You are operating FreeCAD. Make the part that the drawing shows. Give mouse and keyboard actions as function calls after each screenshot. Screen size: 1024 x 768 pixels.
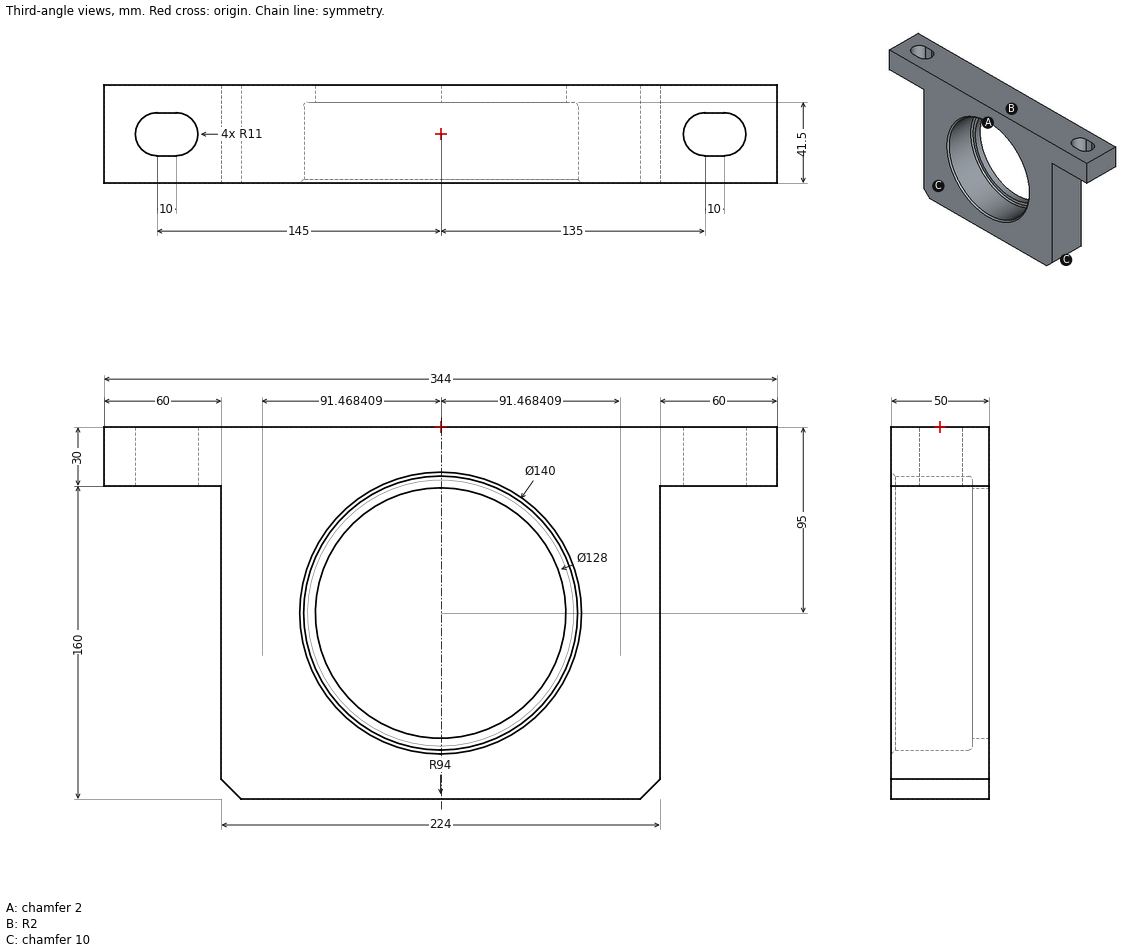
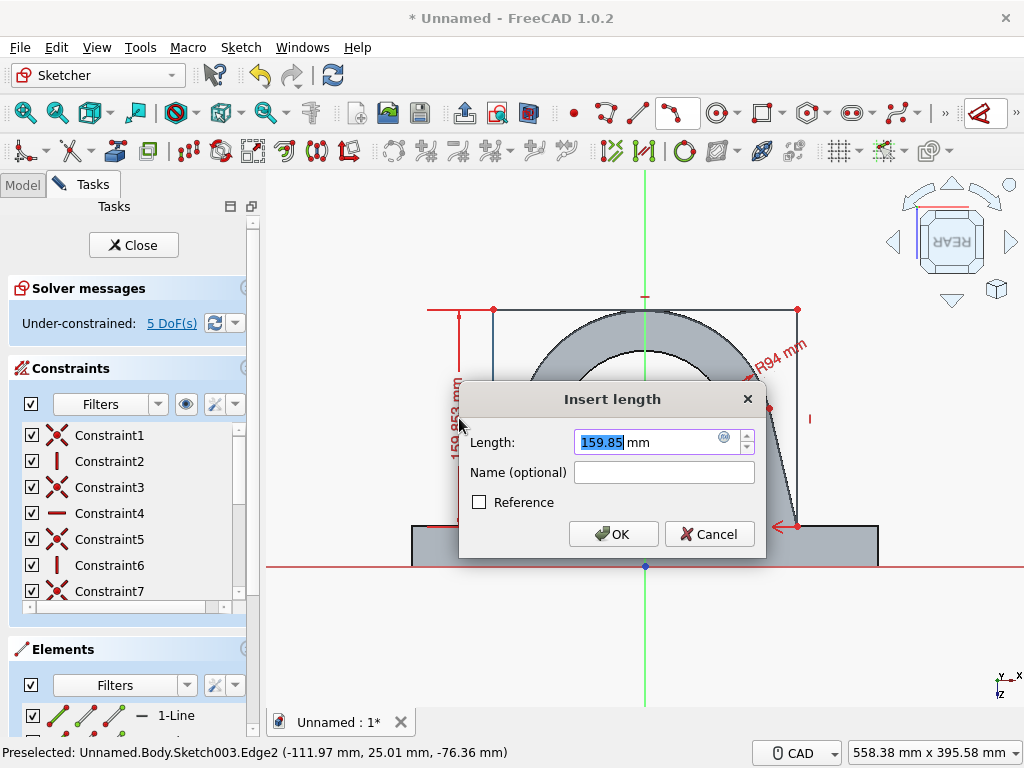
text(160)
key(Return)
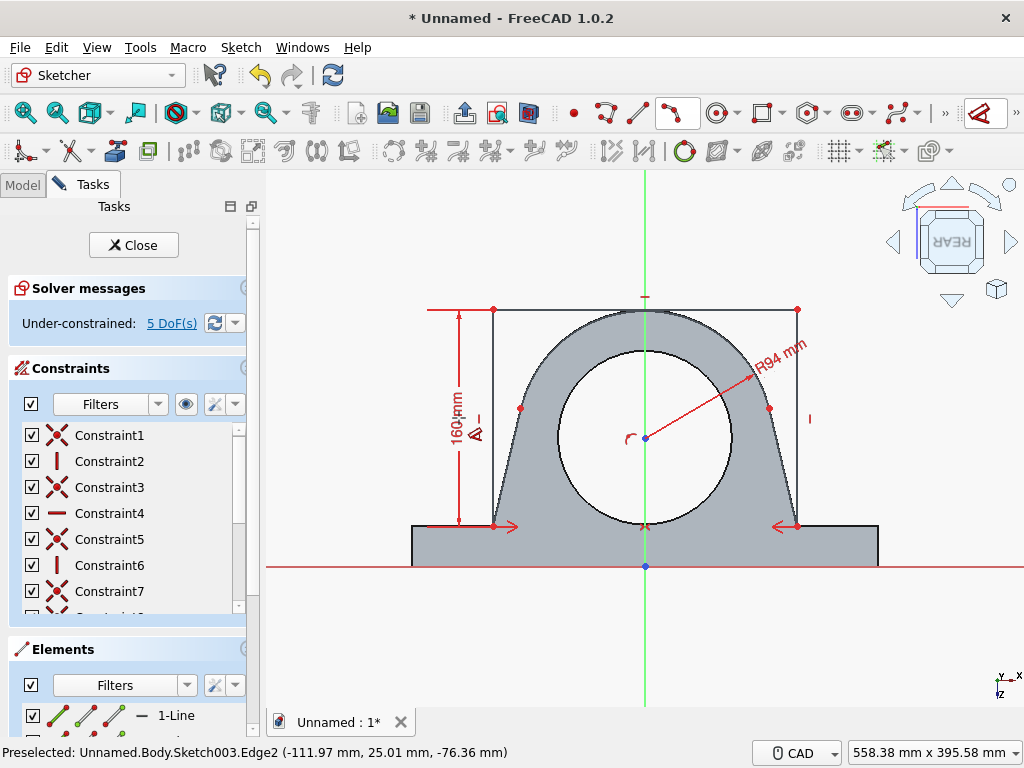
click(584, 310)
click(575, 276)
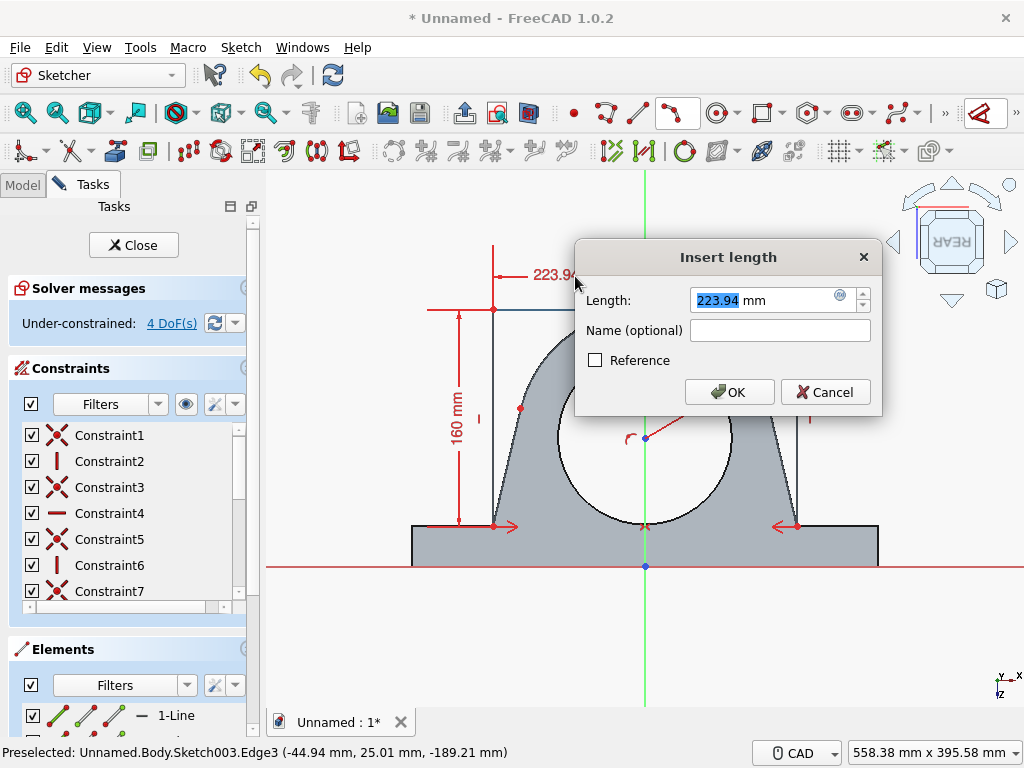
text(224)
key(Return)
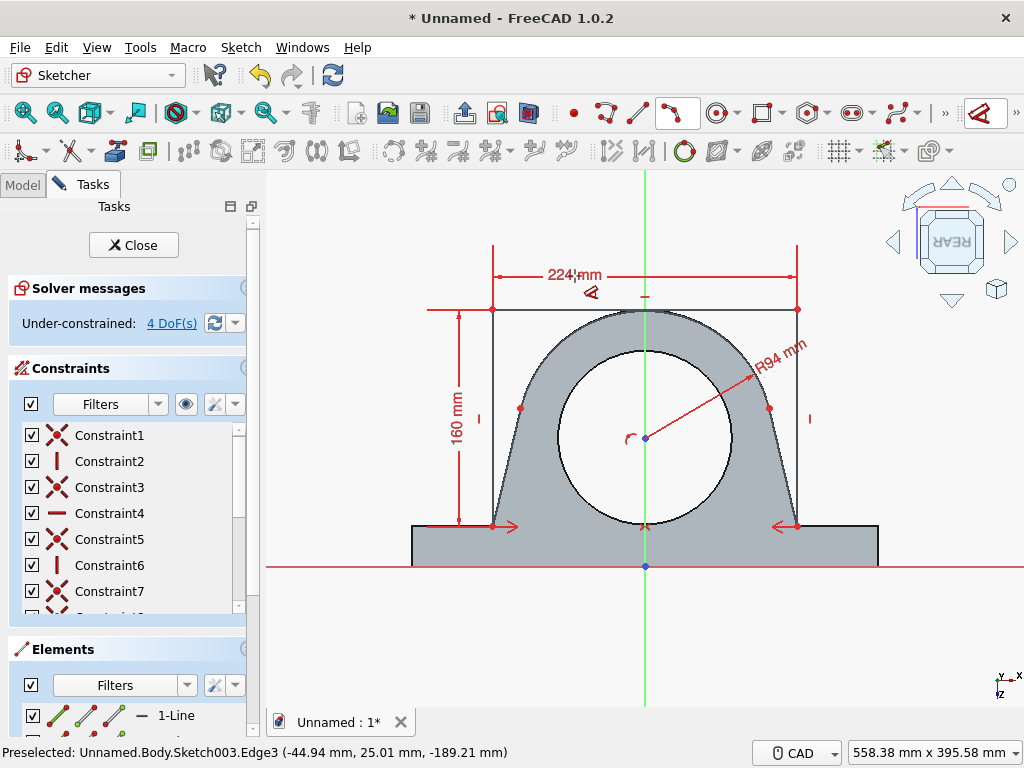
click(493, 527)
click(459, 547)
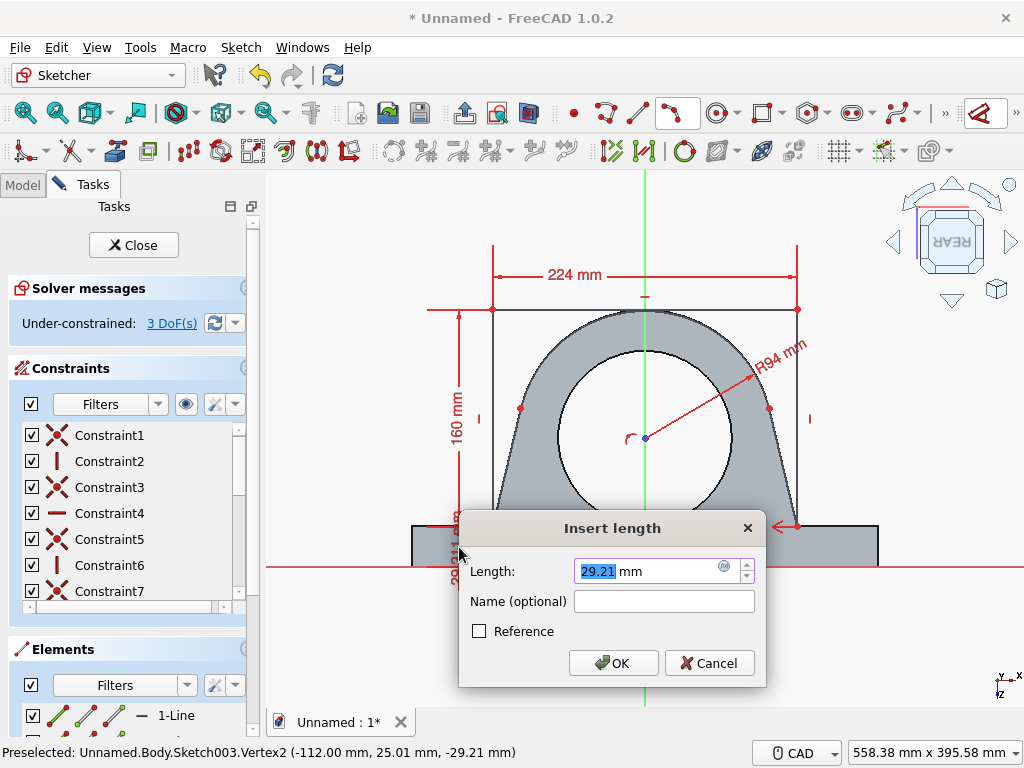
text(30)
key(Return)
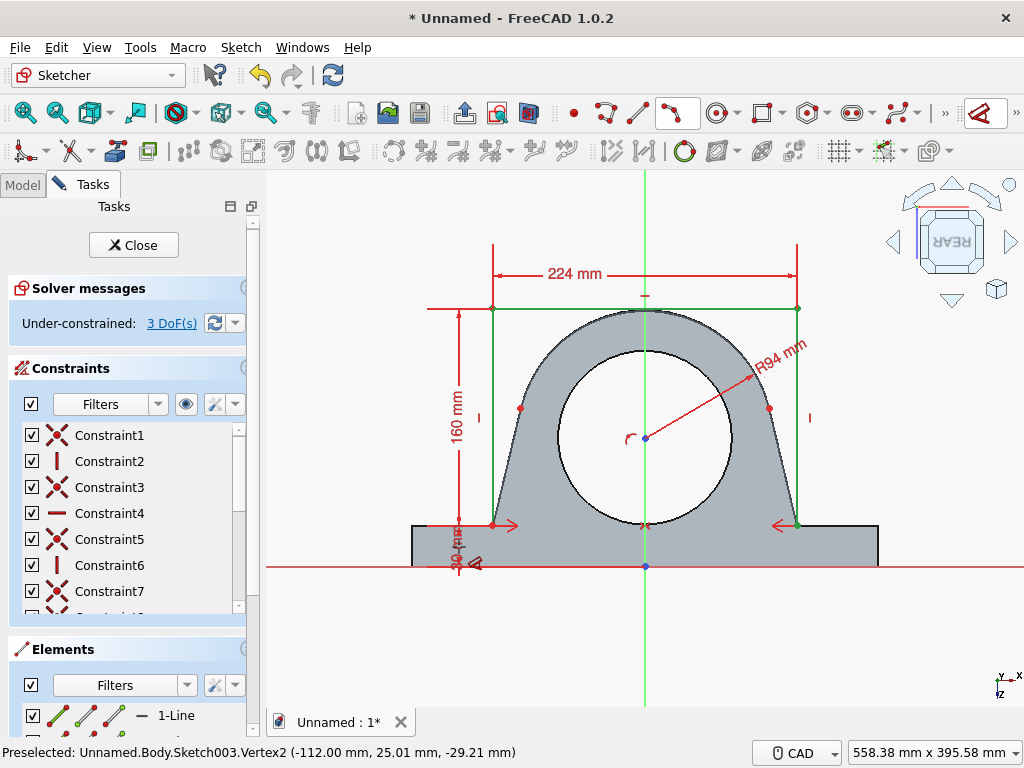
click(645, 439)
click(679, 503)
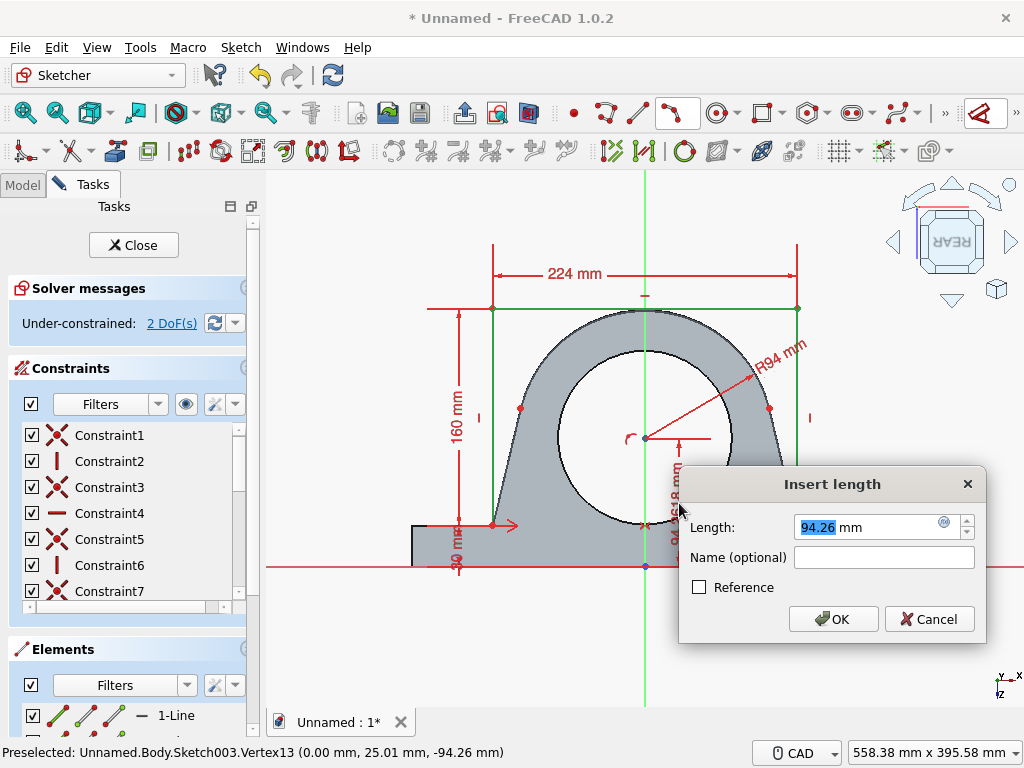
text(95)
key(Return)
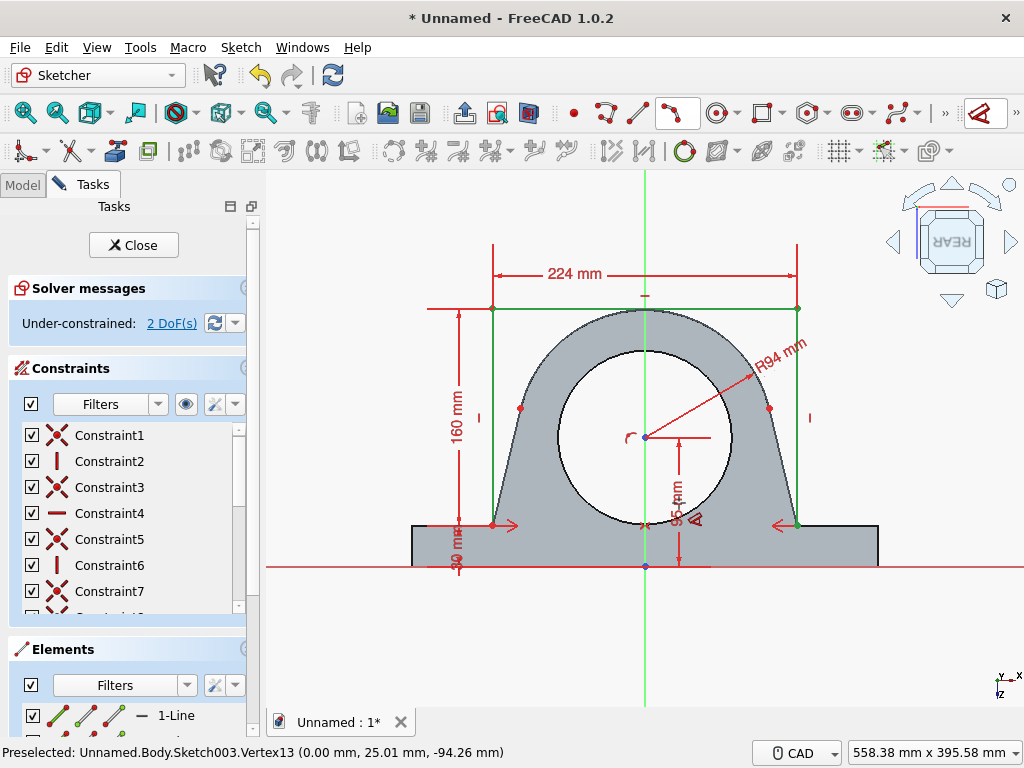
click(521, 409)
click(583, 601)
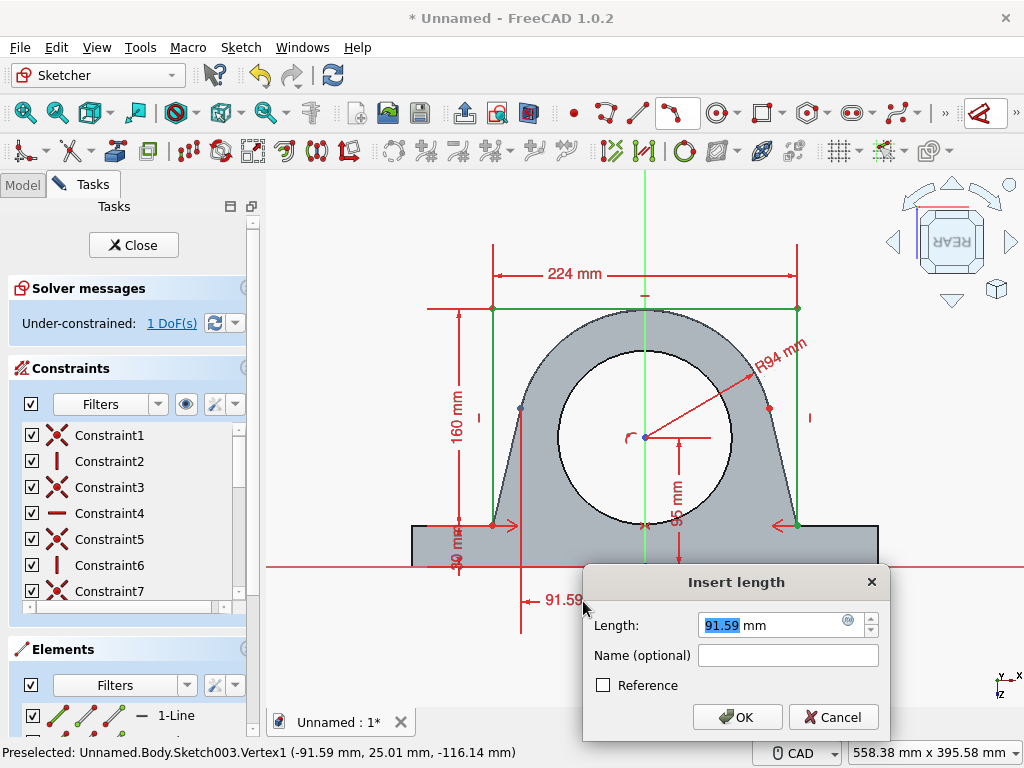
text(91.468409)
key(Return)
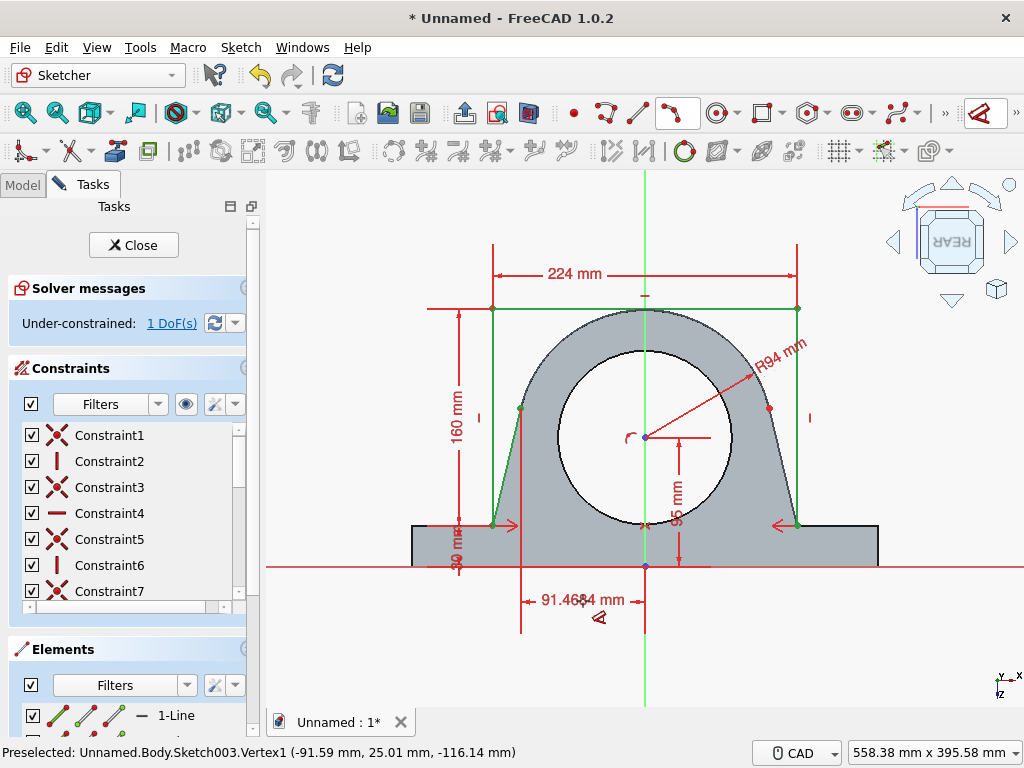
click(769, 409)
click(707, 601)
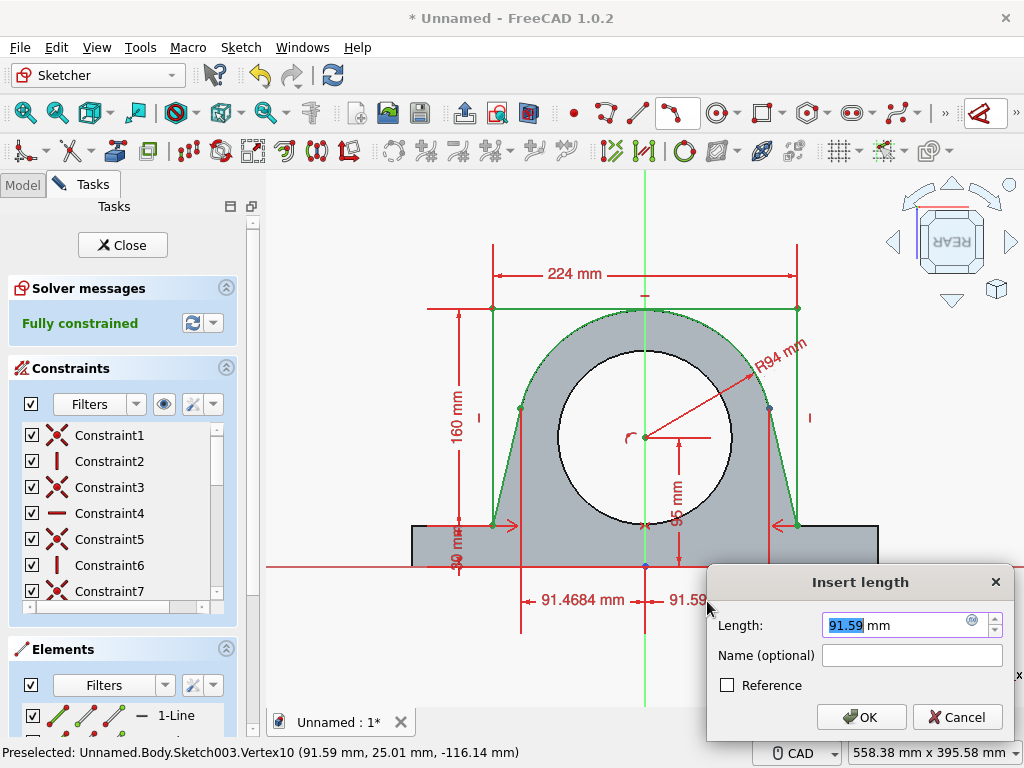
text(91.468409)
key(Return)
key(Escape)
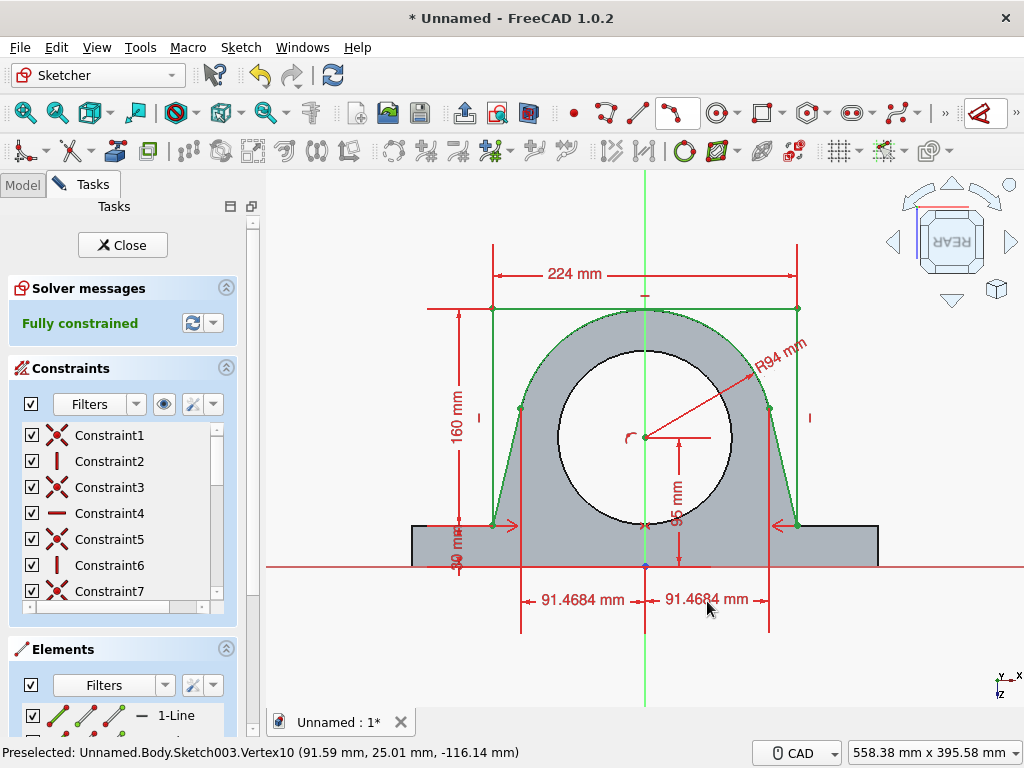
click(123, 245)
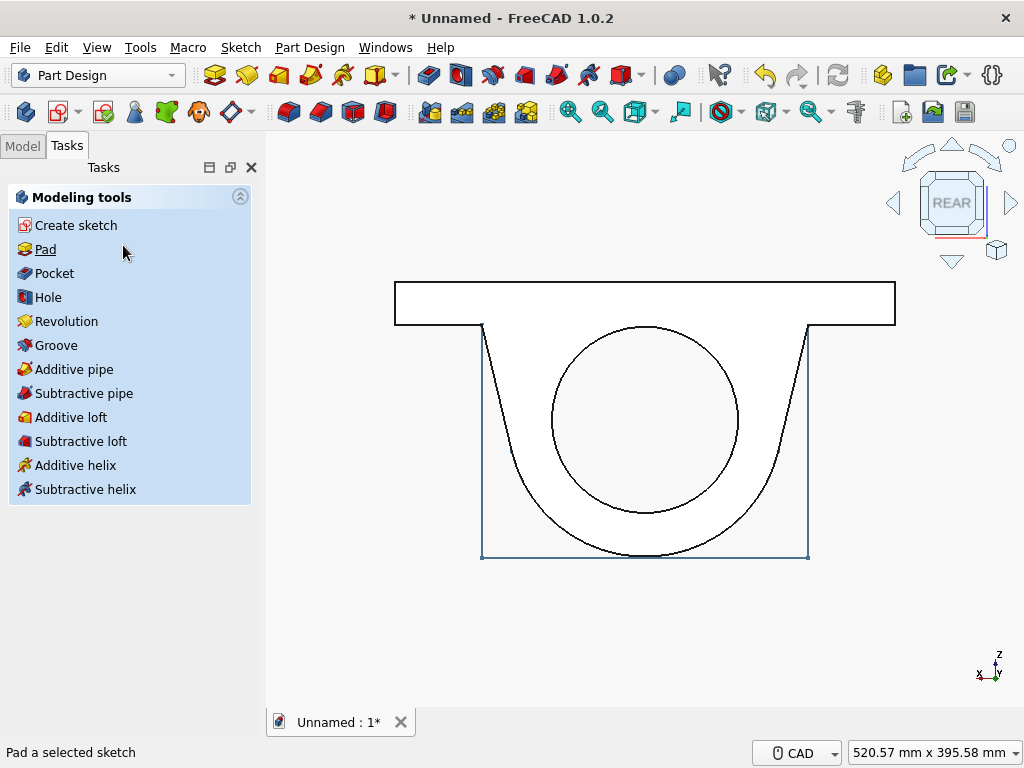
click(216, 76)